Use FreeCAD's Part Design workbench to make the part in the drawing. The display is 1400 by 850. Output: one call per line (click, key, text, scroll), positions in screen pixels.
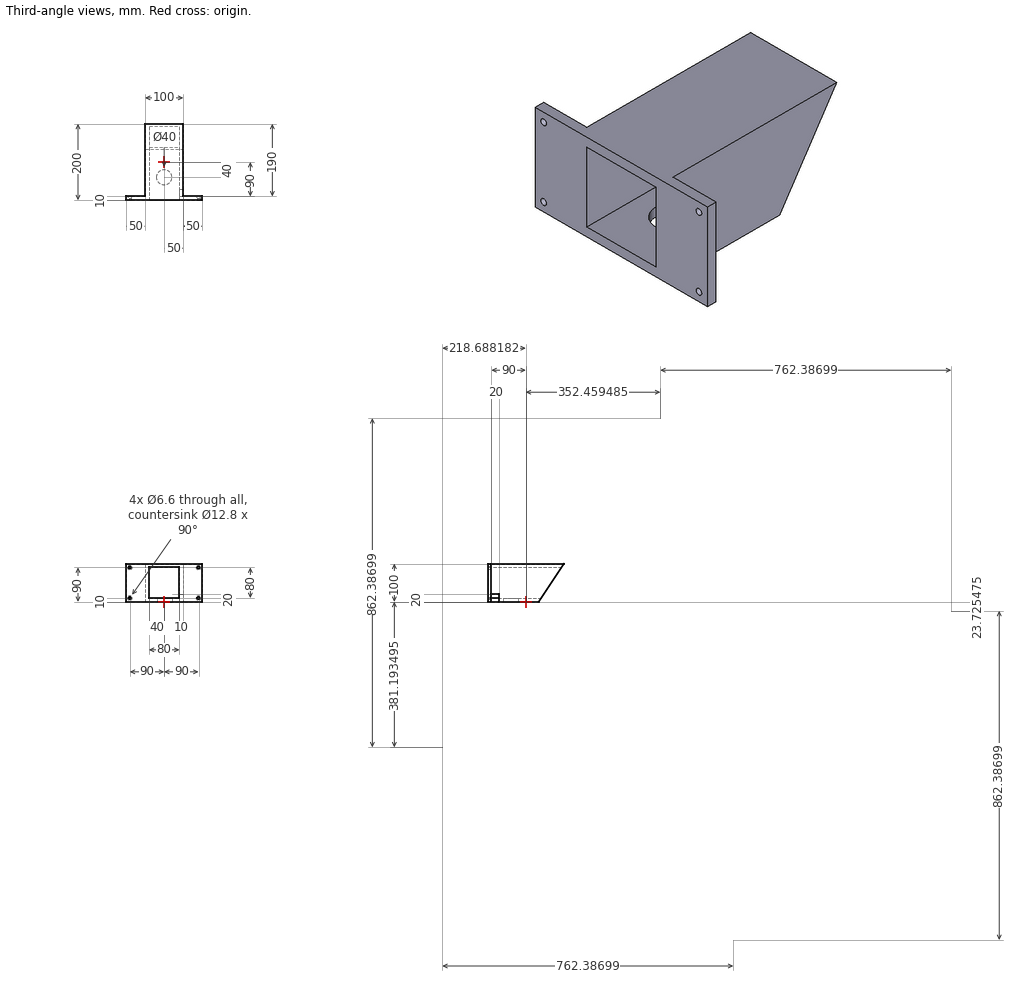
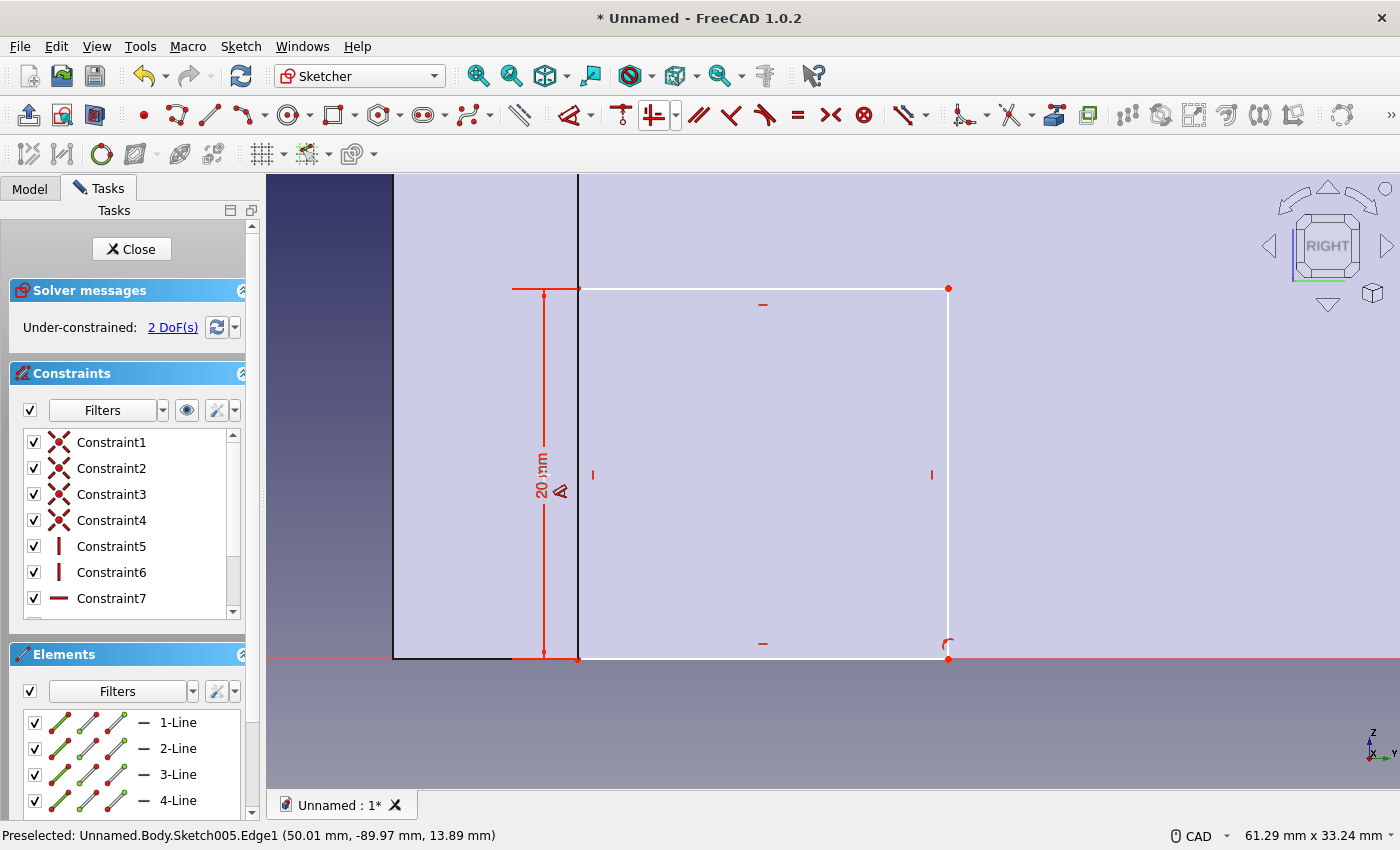
click(689, 659)
click(763, 693)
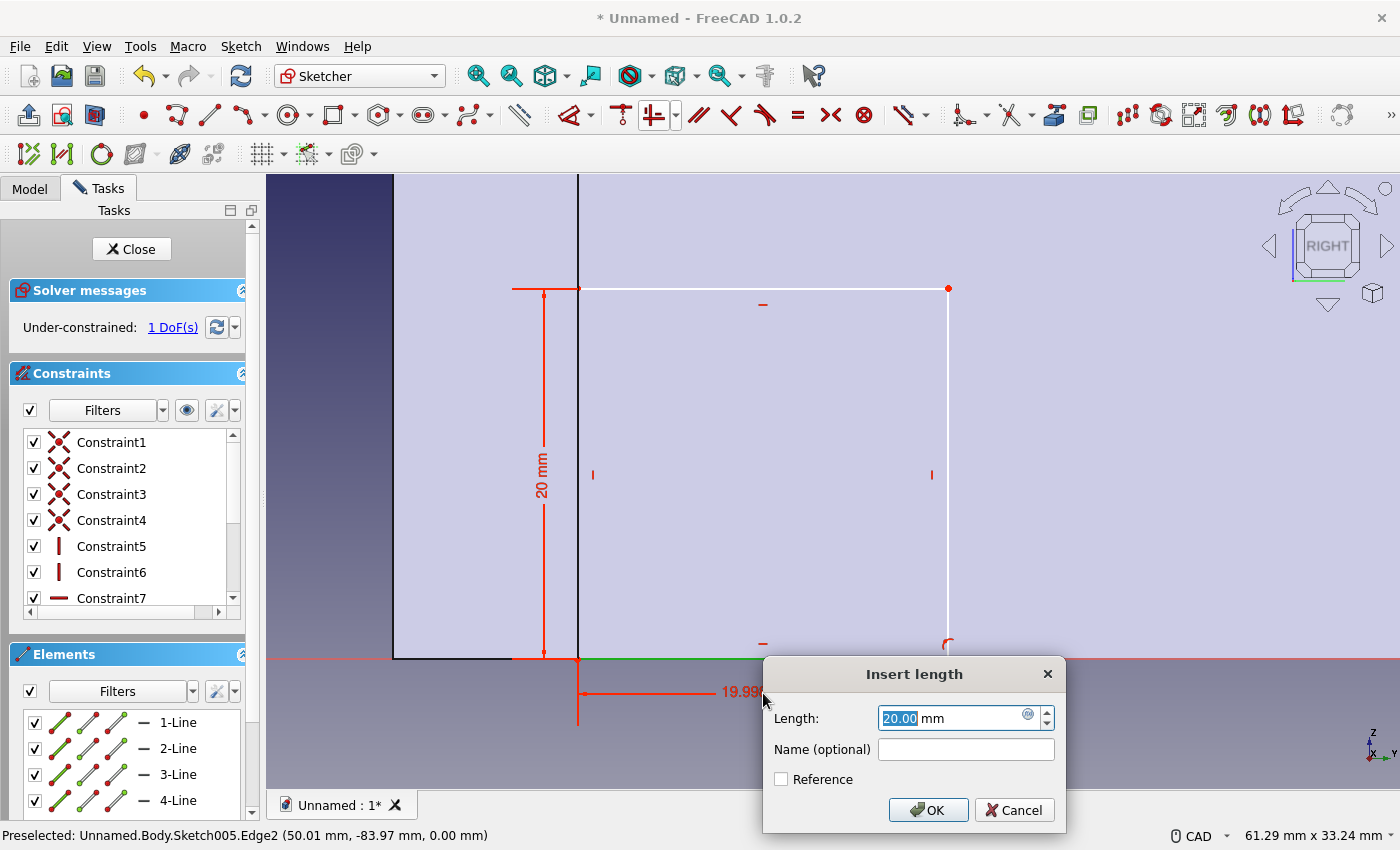
text(20)
key(Return)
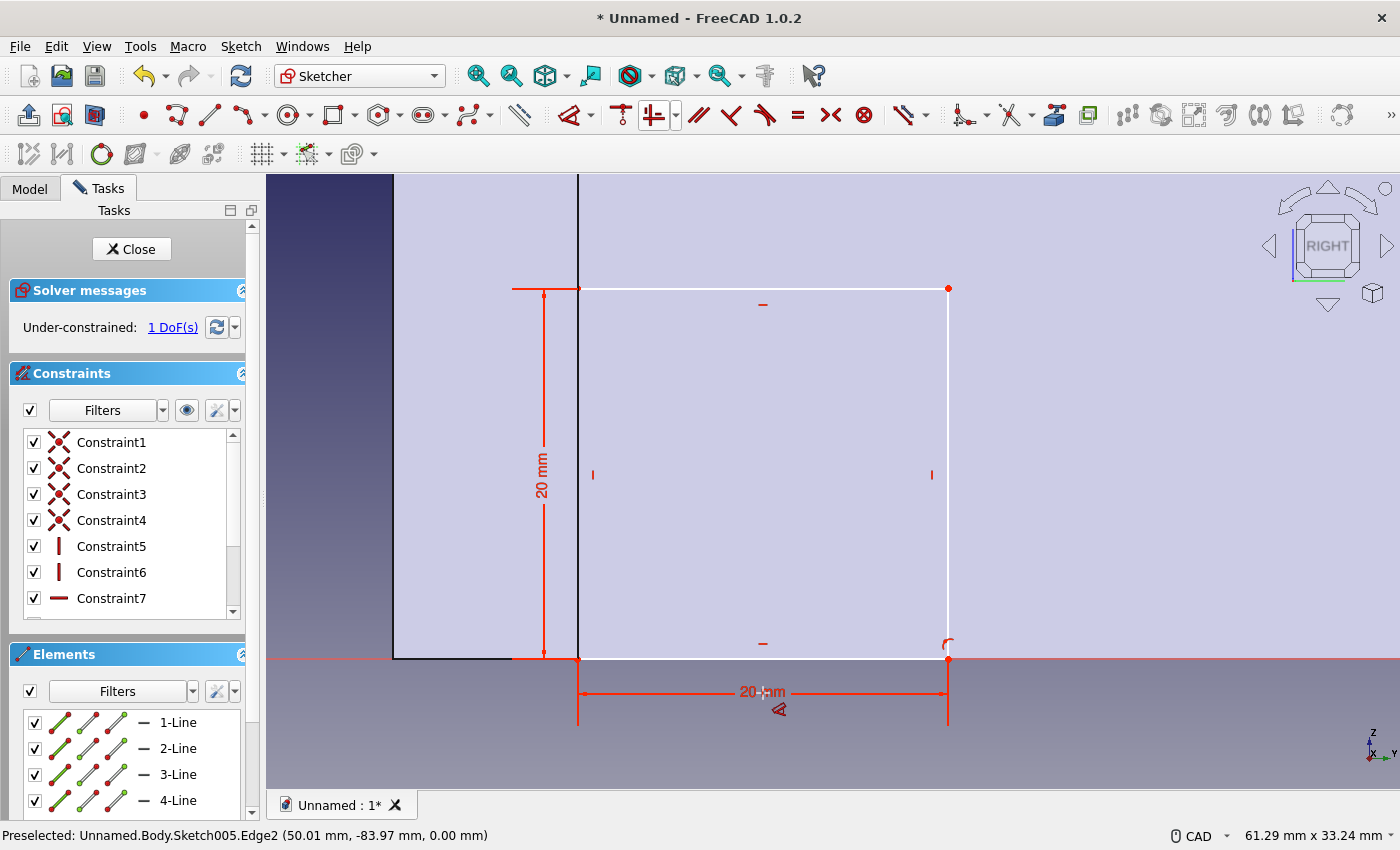
click(578, 289)
click(907, 693)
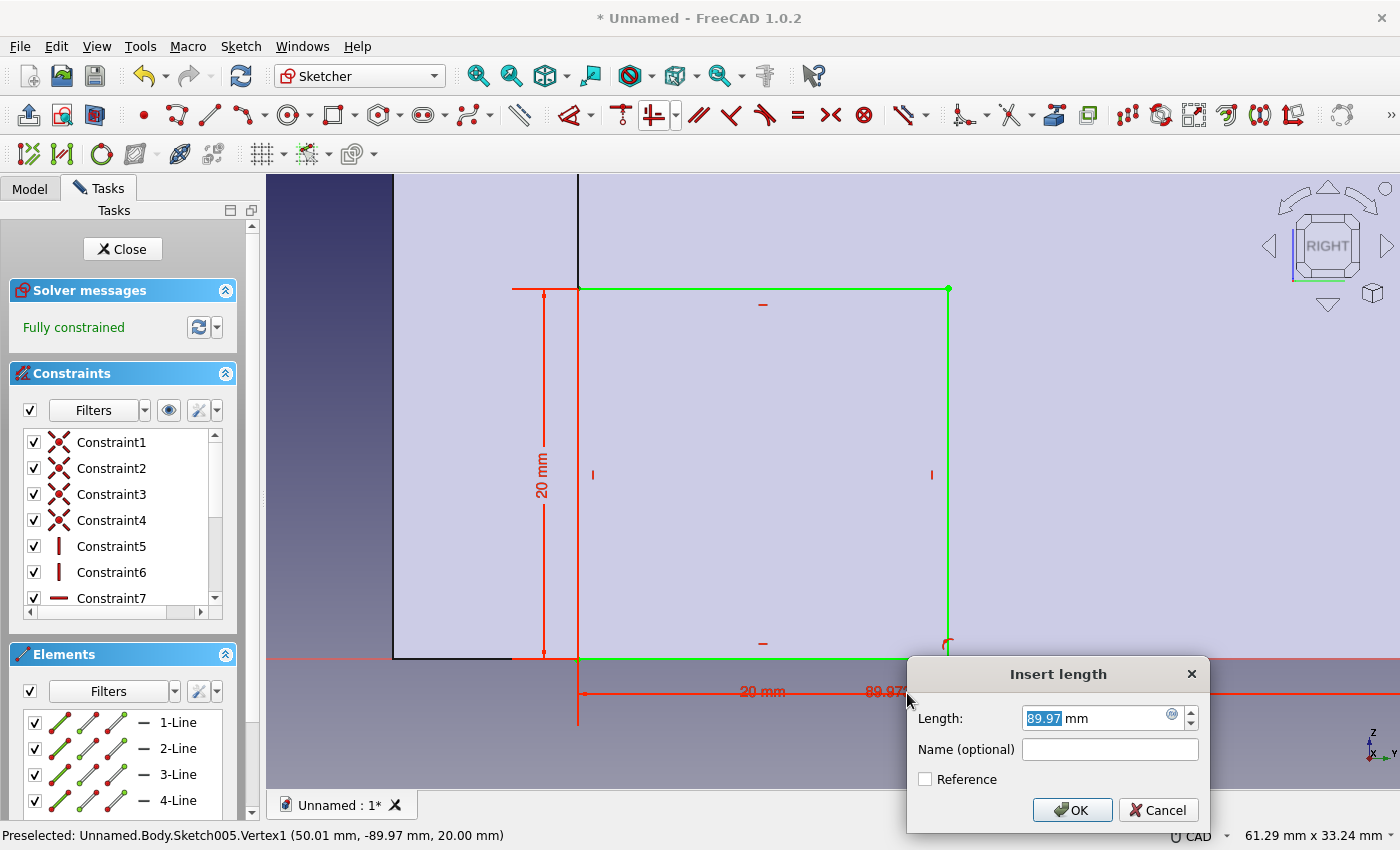
text(90)
key(Return)
key(Escape)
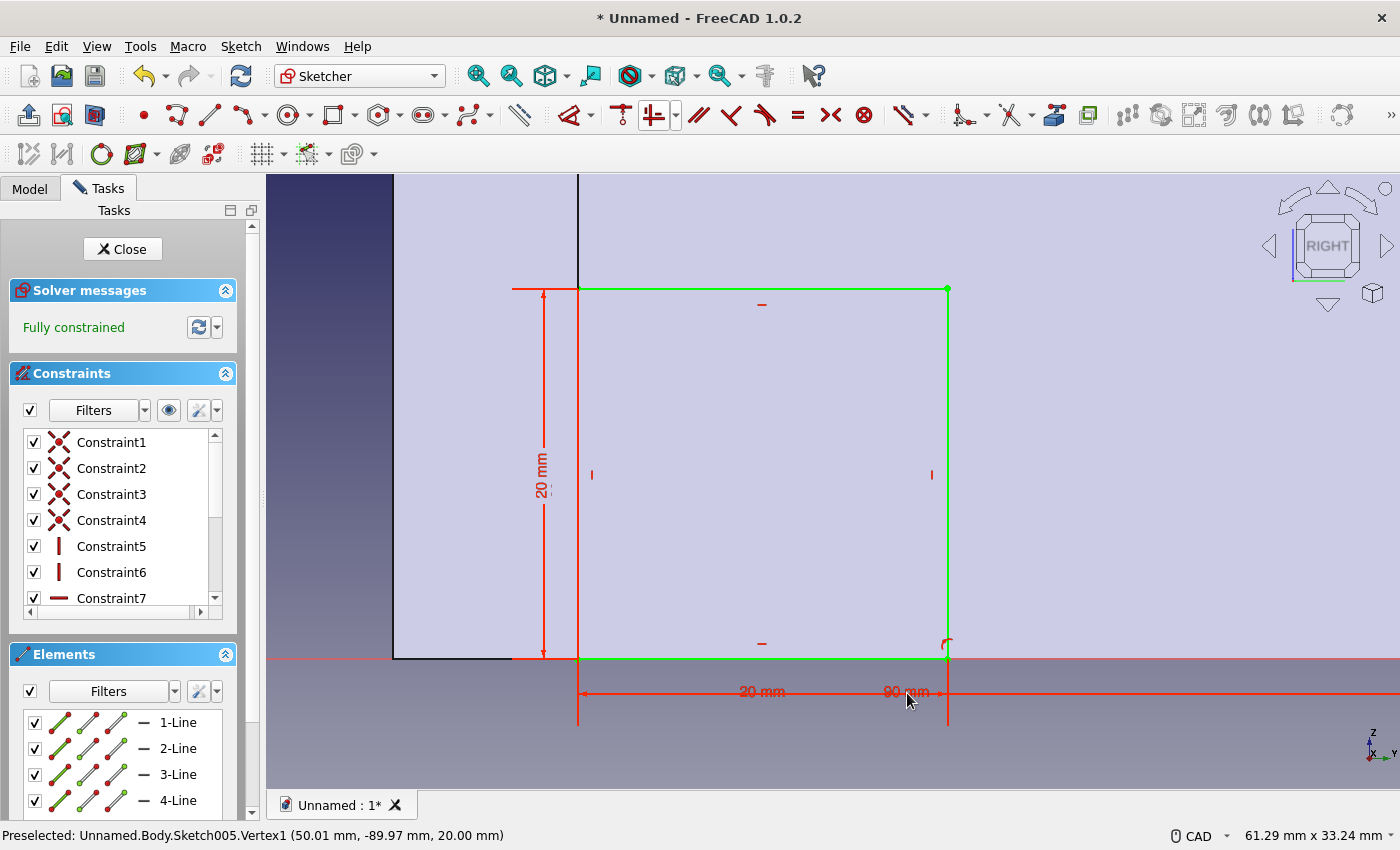
click(123, 249)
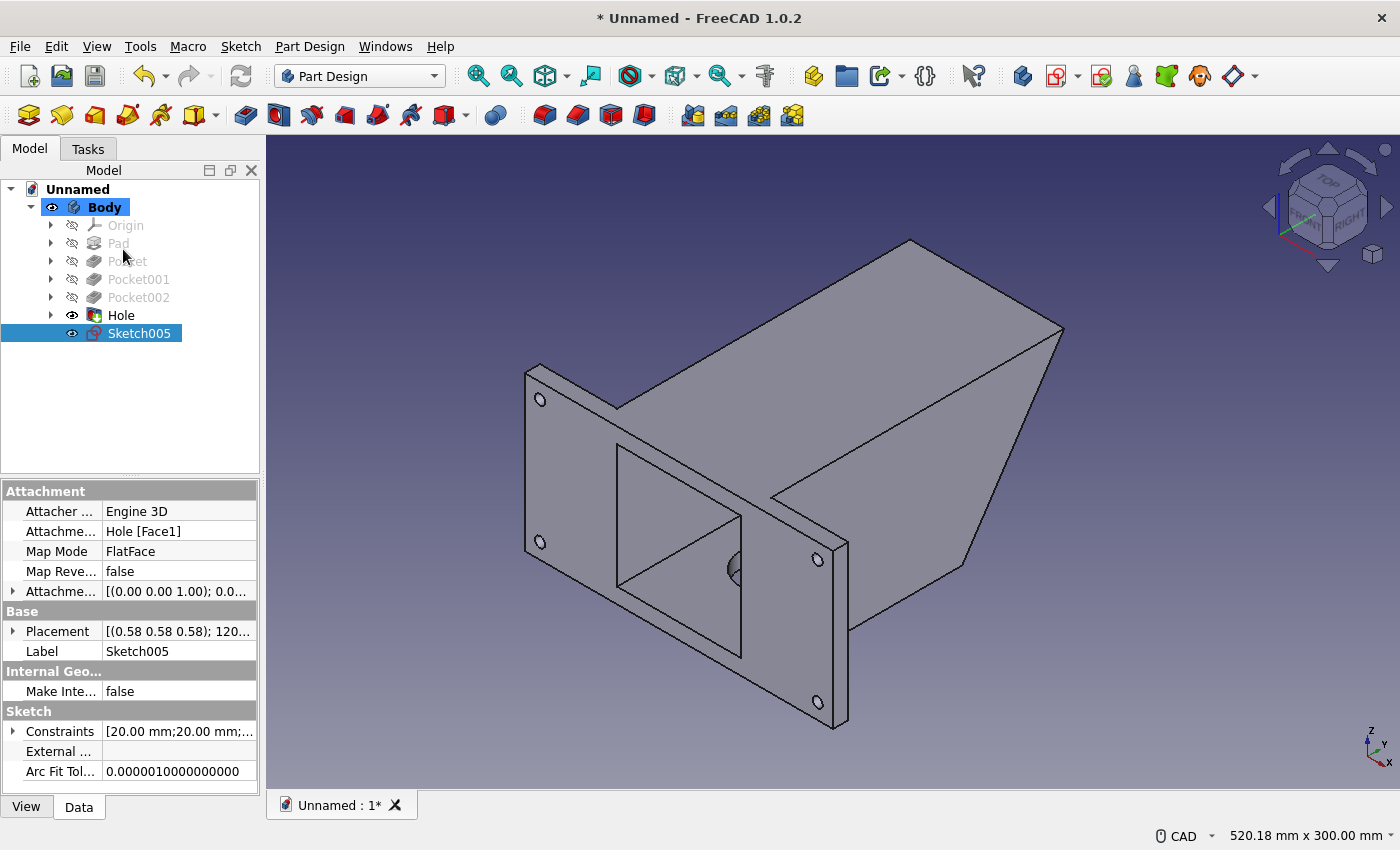
click(246, 116)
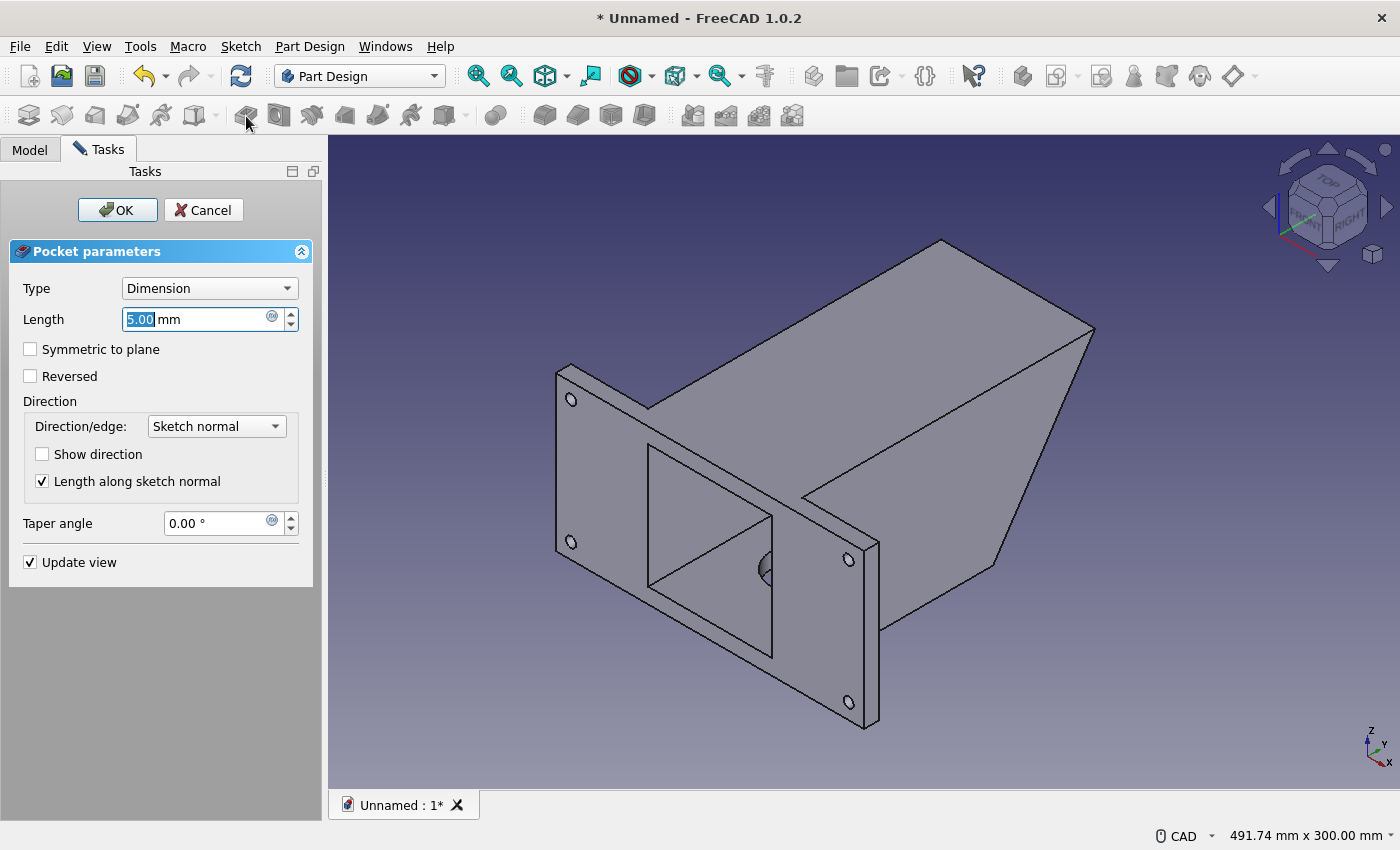
text(10)
key(Tab)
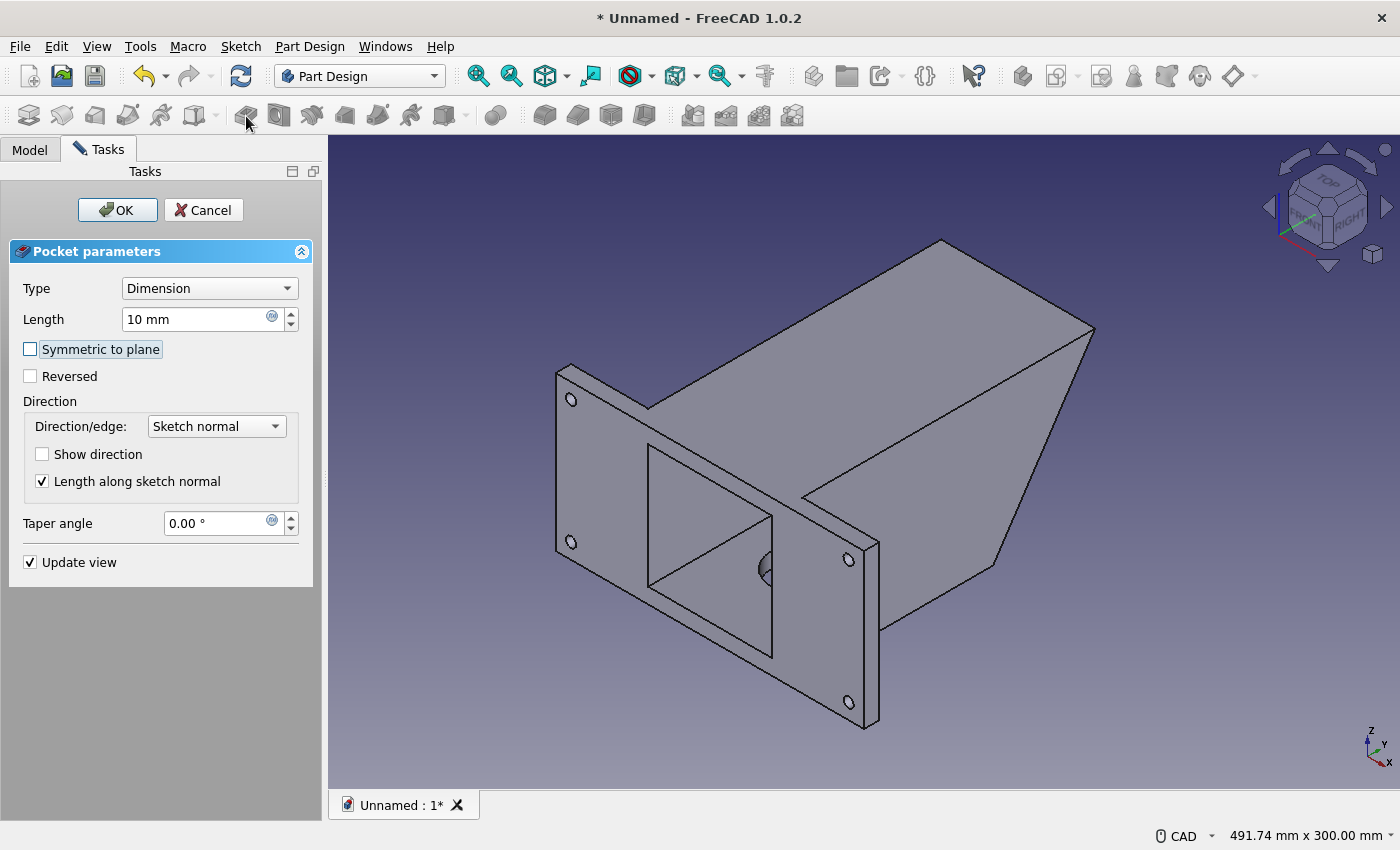
click(118, 210)